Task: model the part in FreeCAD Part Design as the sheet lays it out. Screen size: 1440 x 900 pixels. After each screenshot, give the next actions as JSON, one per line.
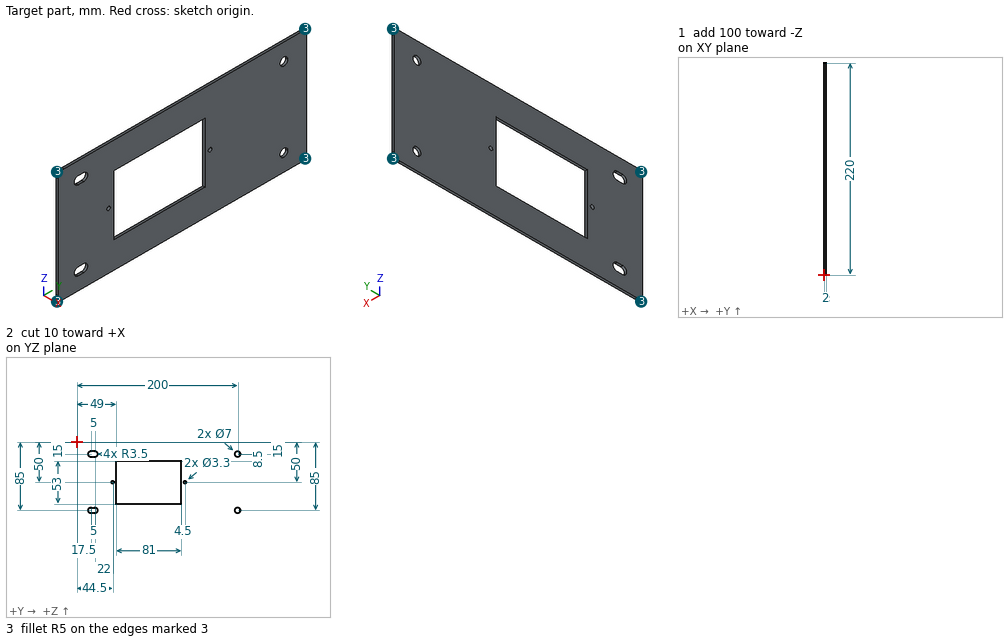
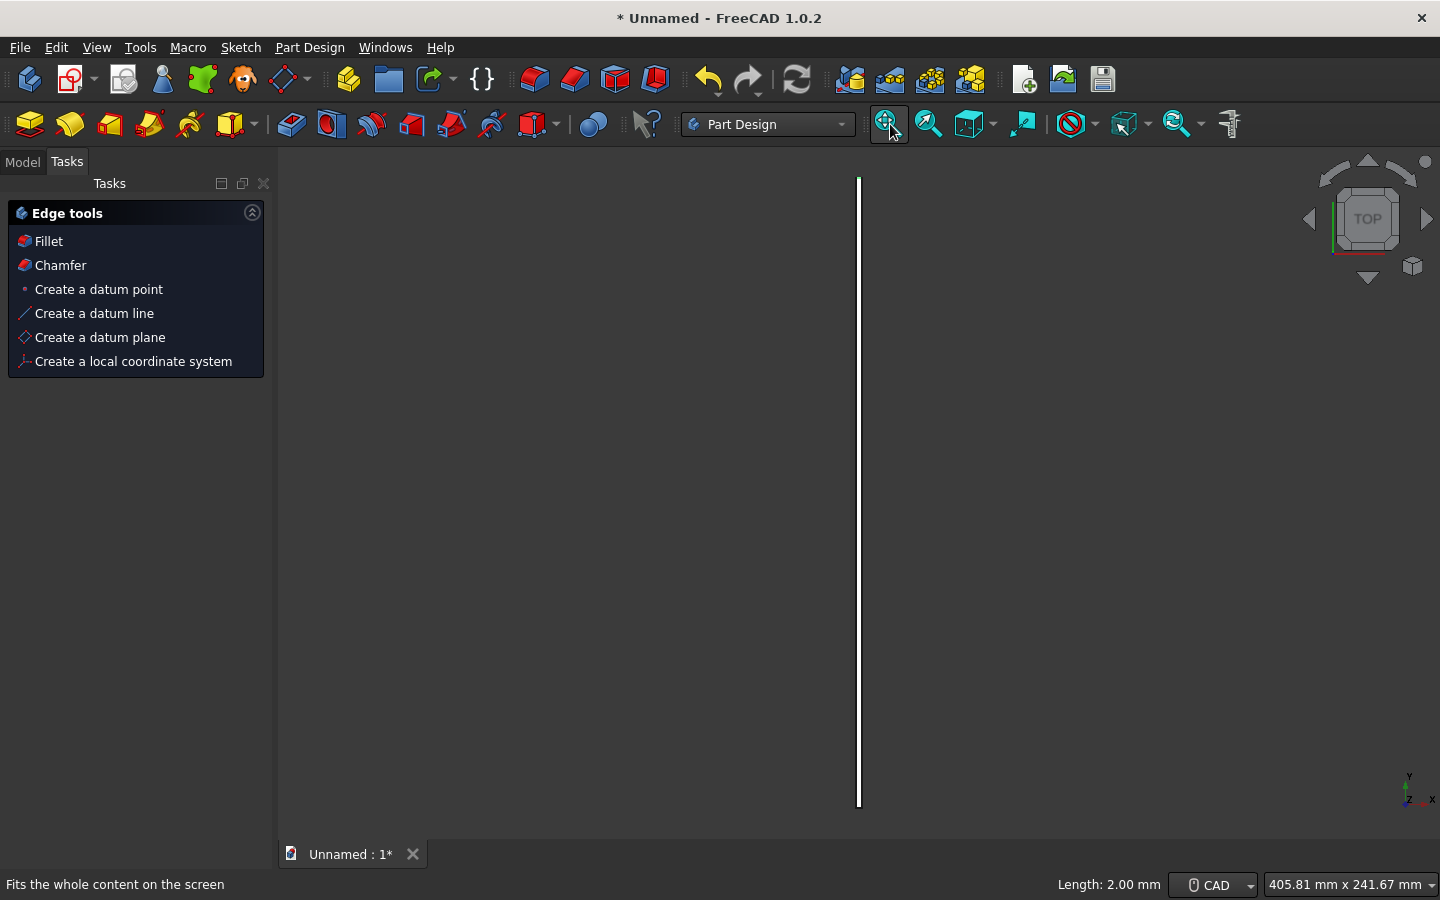
{"action": "key", "text": "1"}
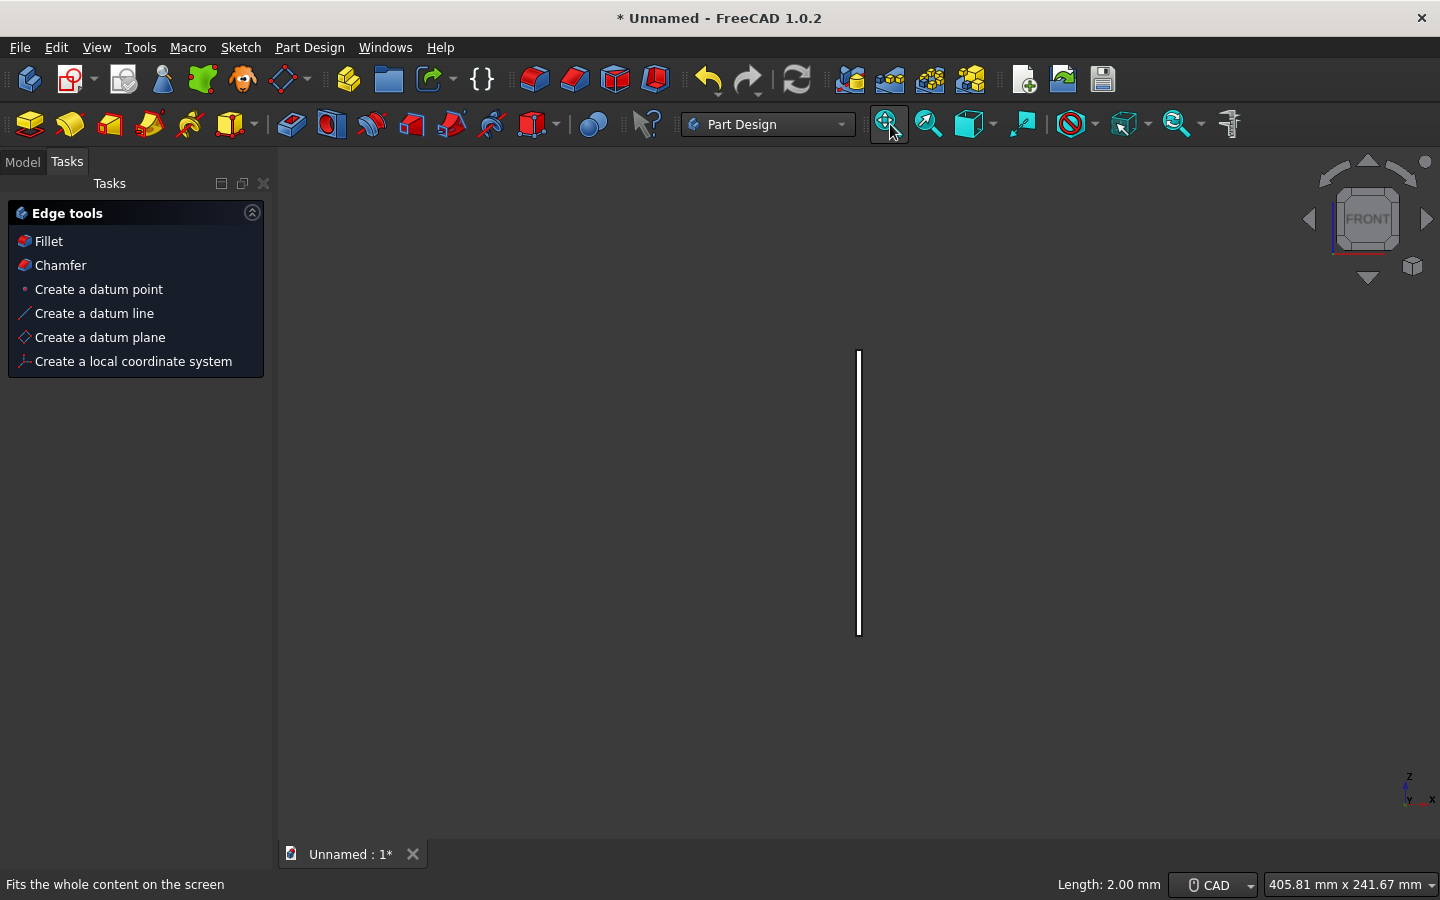
{"action": "left_click", "coordinate": [890, 124]}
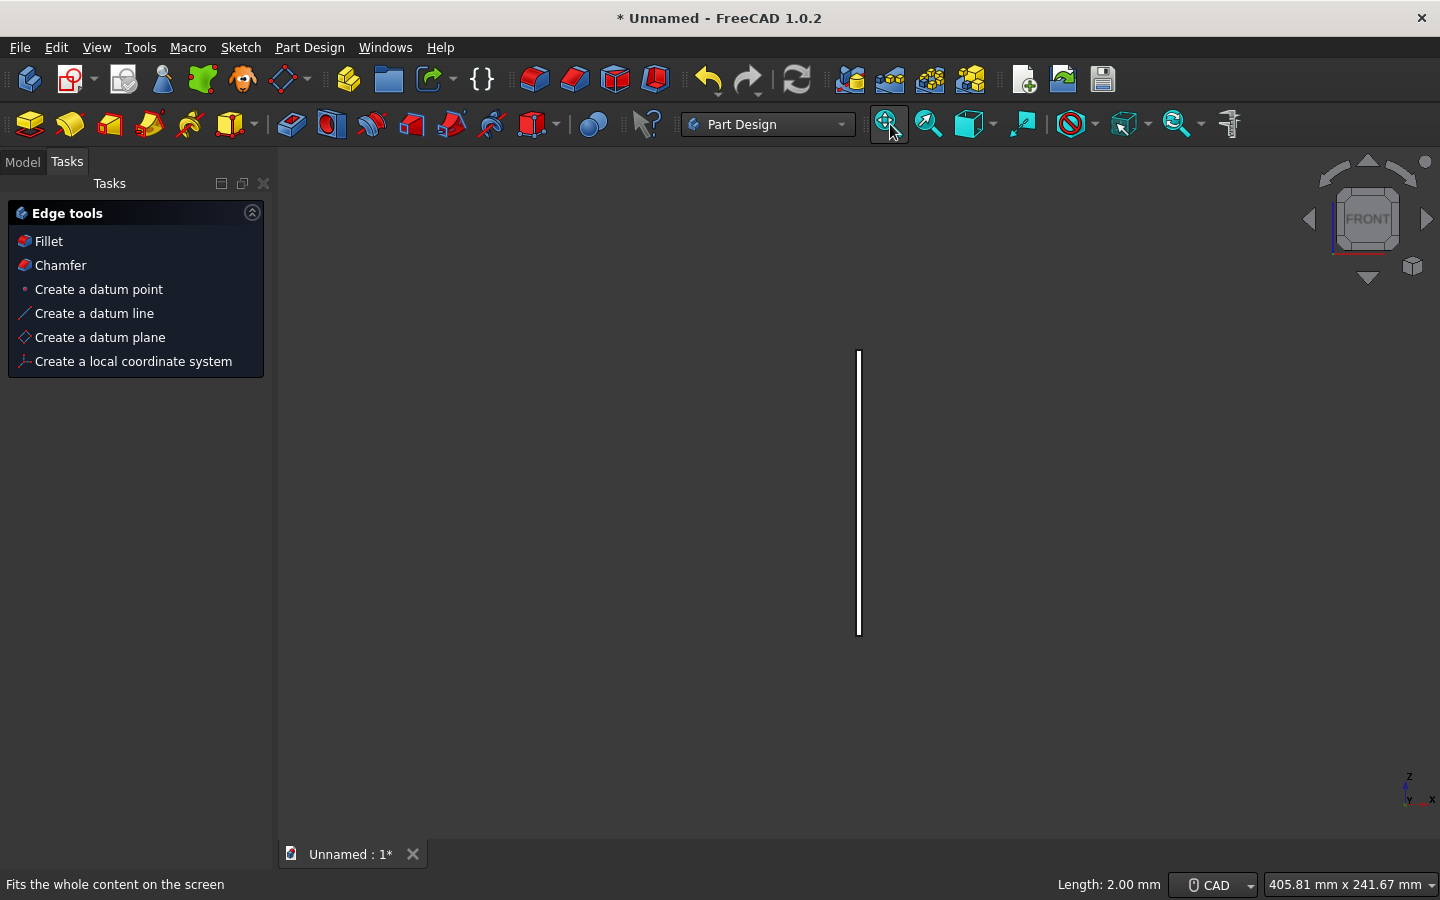
{"action": "scroll", "coordinate": [859, 635], "scroll_direction": "up", "scroll_amount": 10}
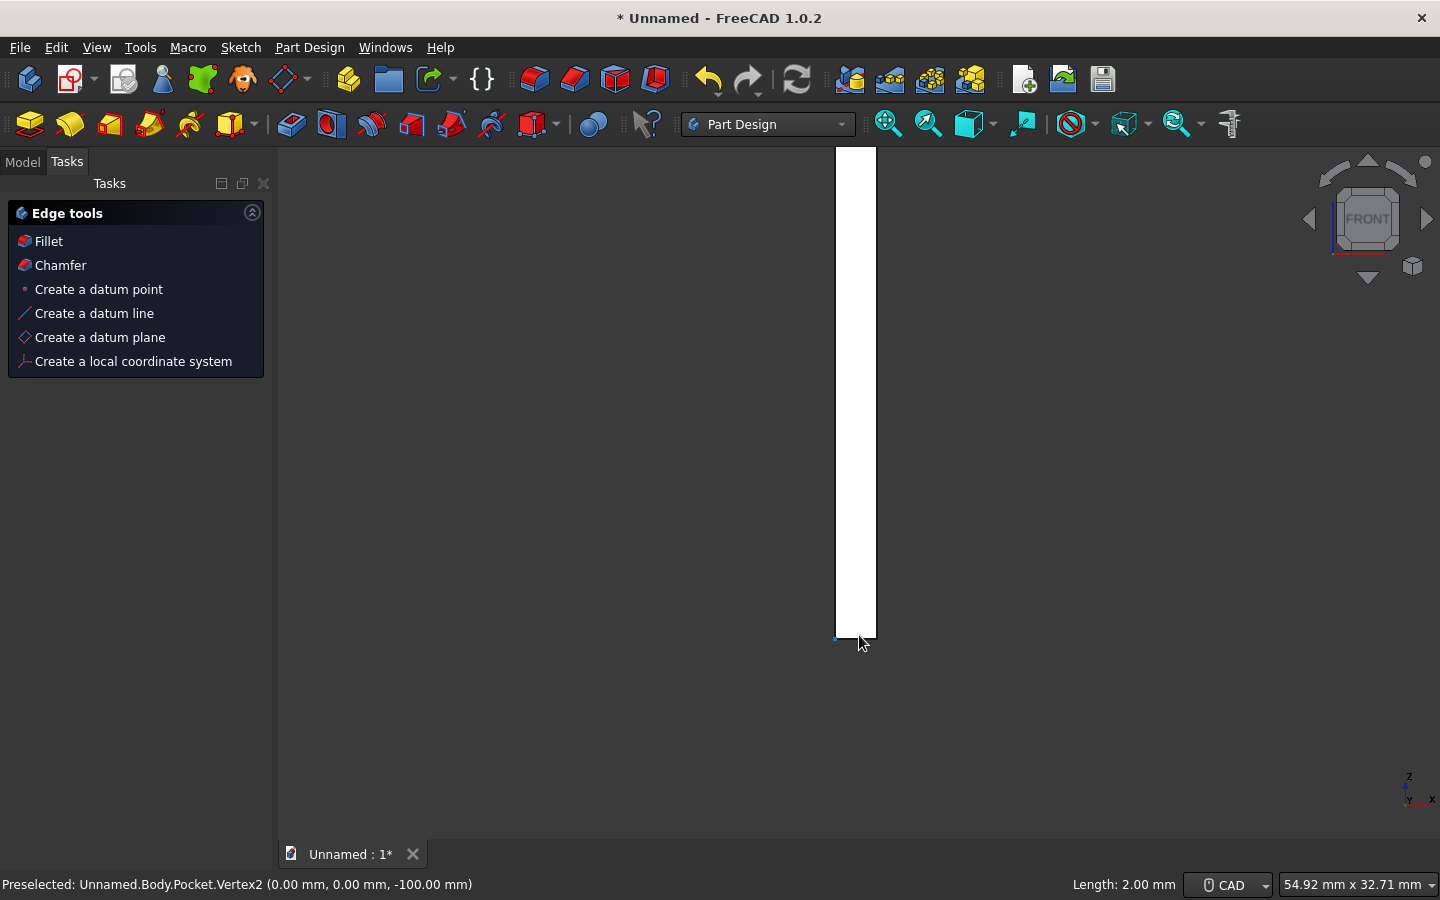
{"action": "left_click", "coordinate": [856, 638], "text": "ctrl"}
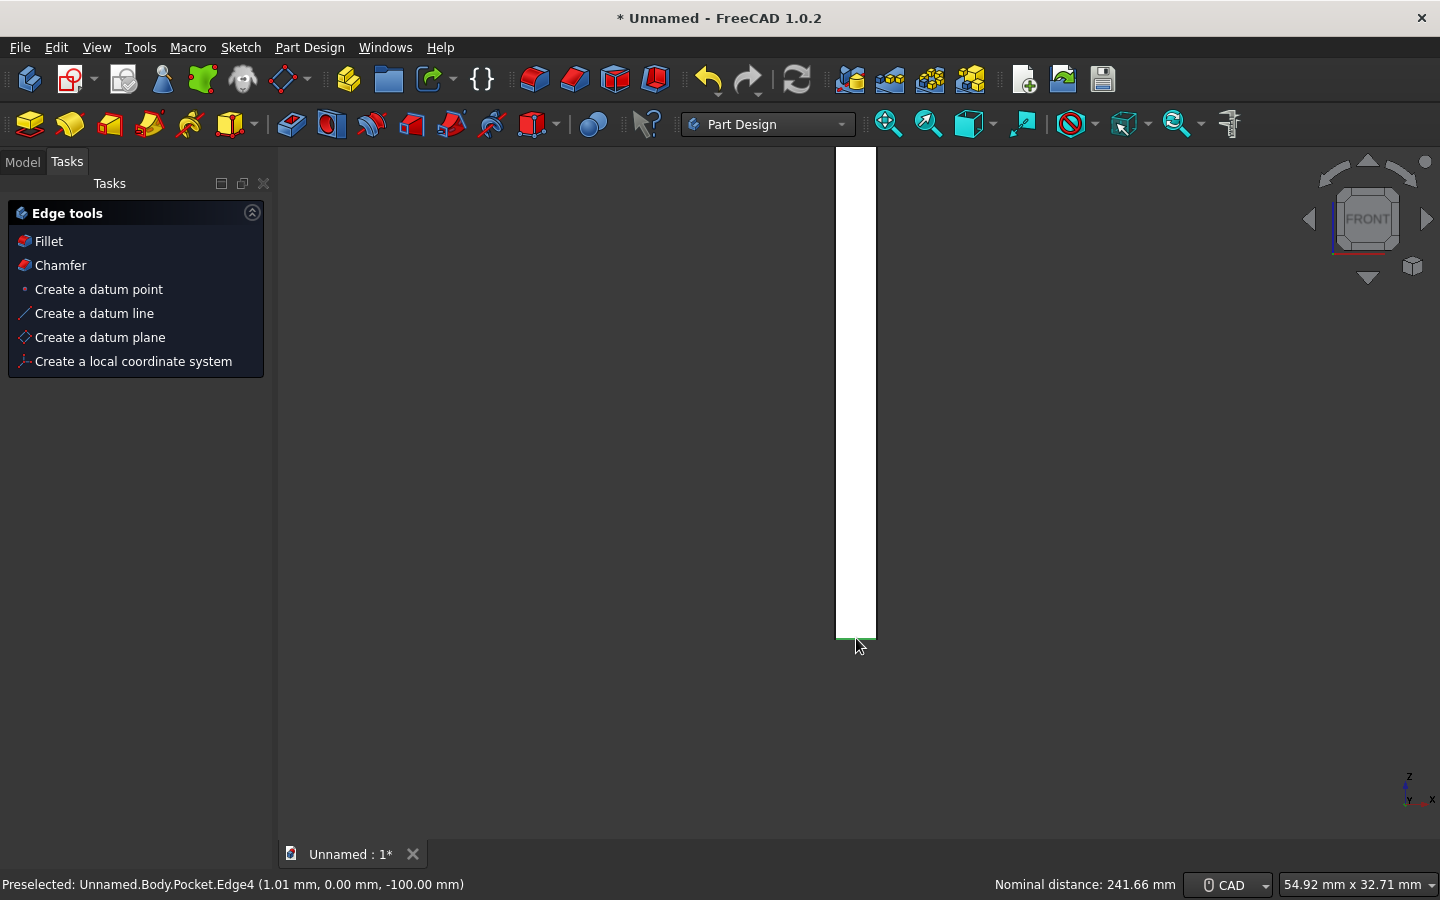
{"action": "left_click", "coordinate": [890, 124]}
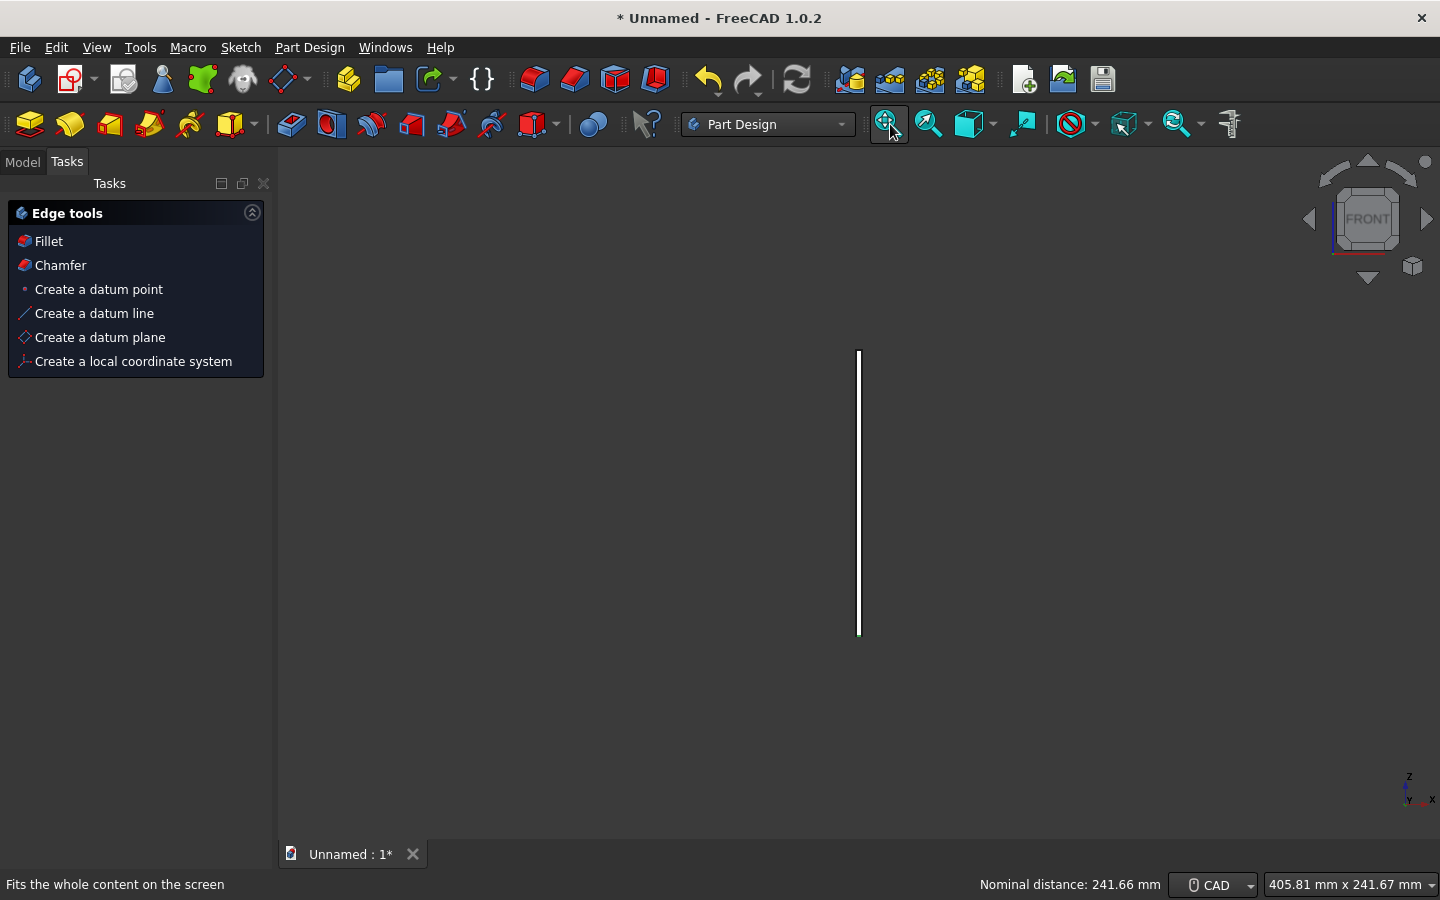
{"action": "key", "text": "3"}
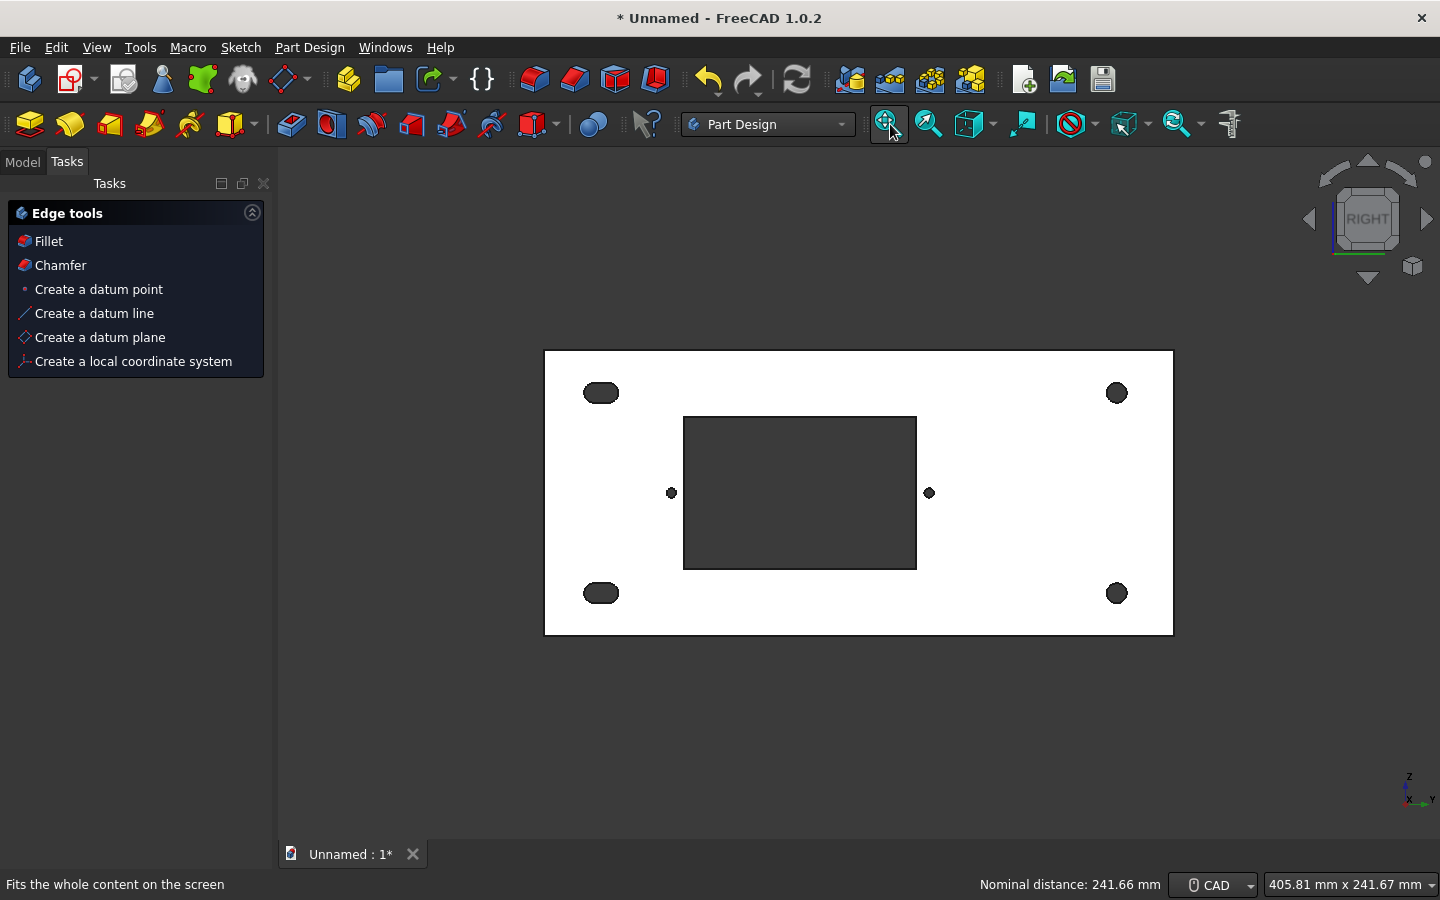
{"action": "scroll", "coordinate": [1174, 635], "scroll_direction": "up", "scroll_amount": 10}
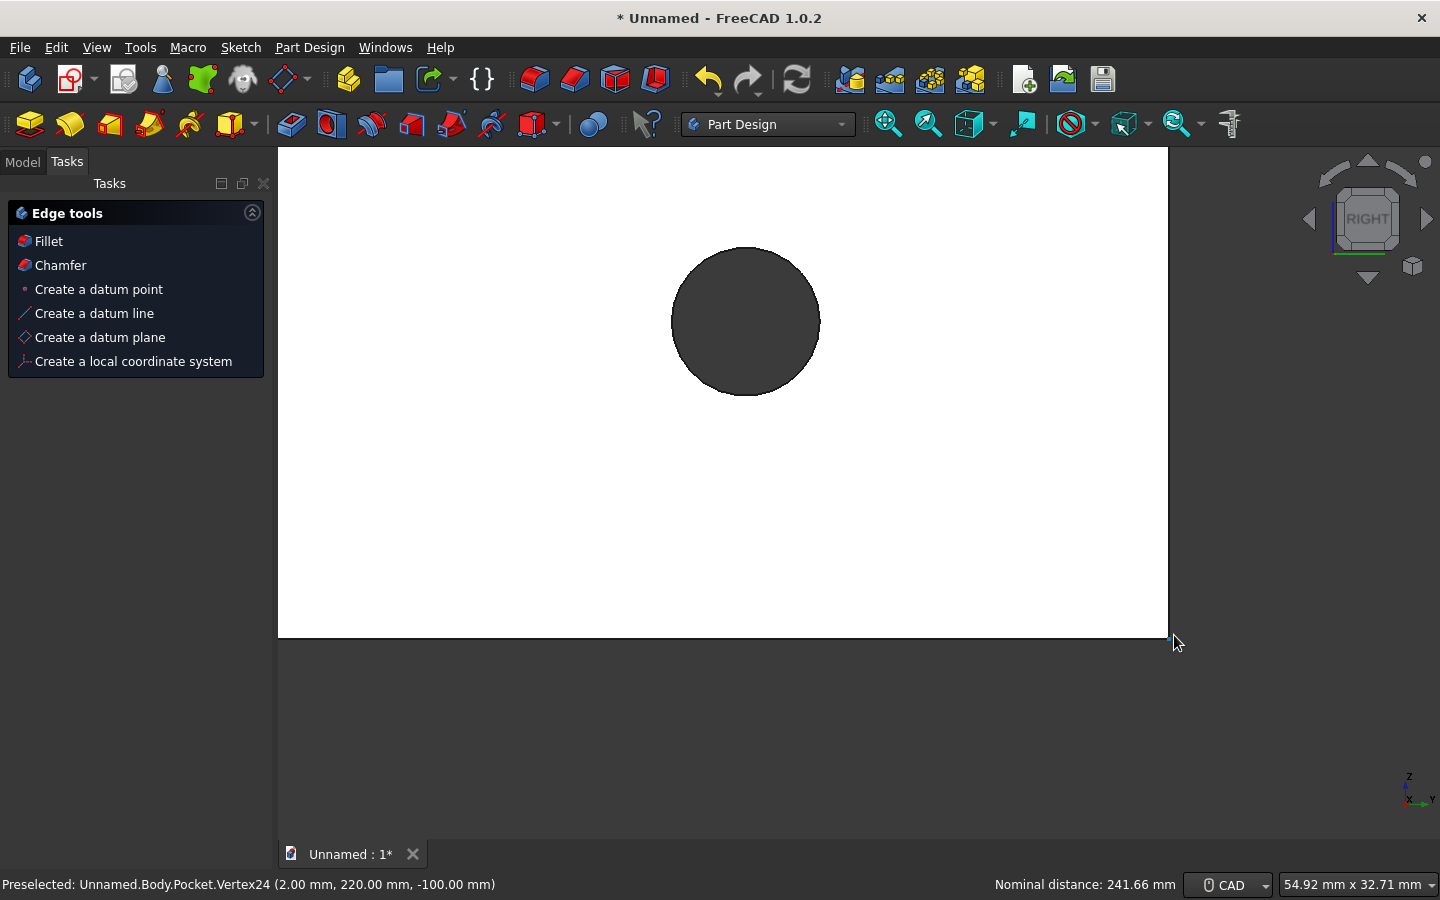
{"action": "left_click", "coordinate": [890, 124]}